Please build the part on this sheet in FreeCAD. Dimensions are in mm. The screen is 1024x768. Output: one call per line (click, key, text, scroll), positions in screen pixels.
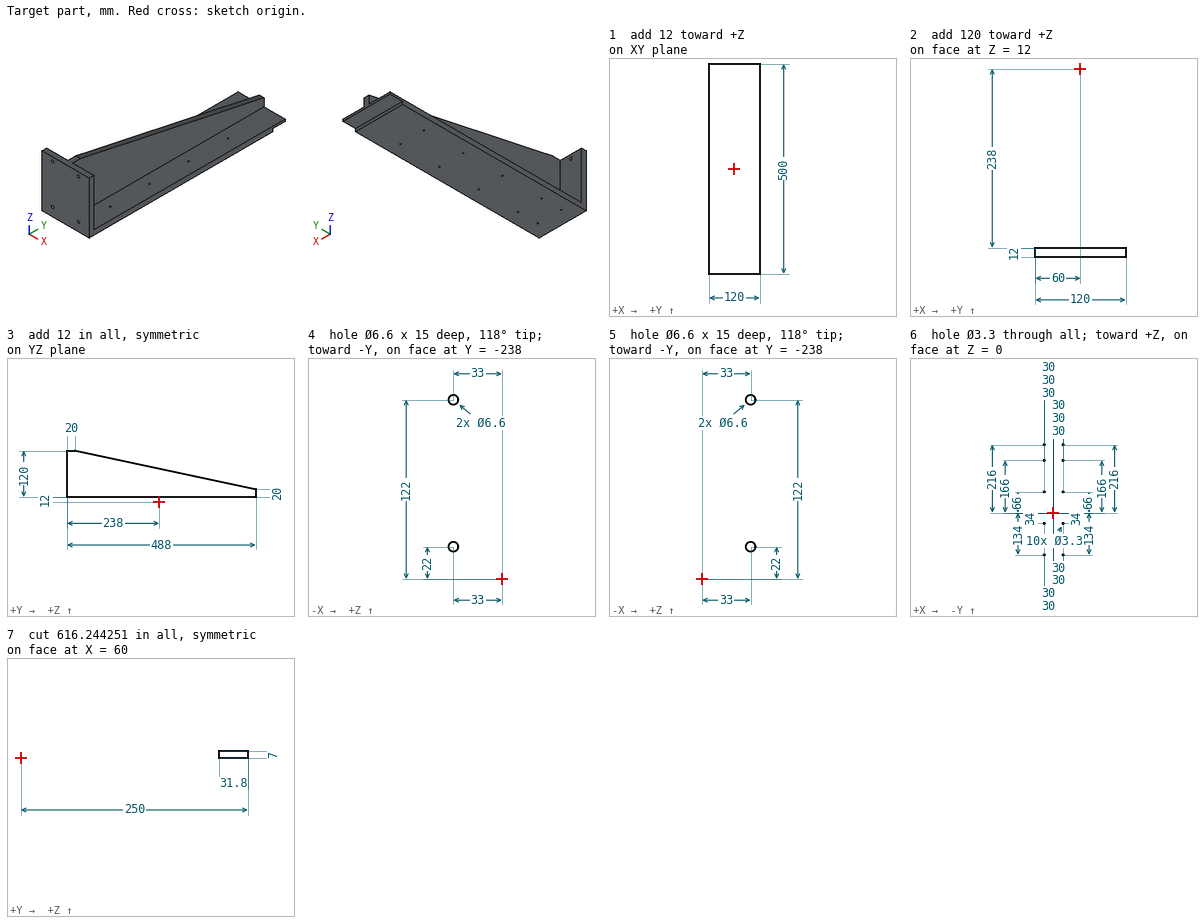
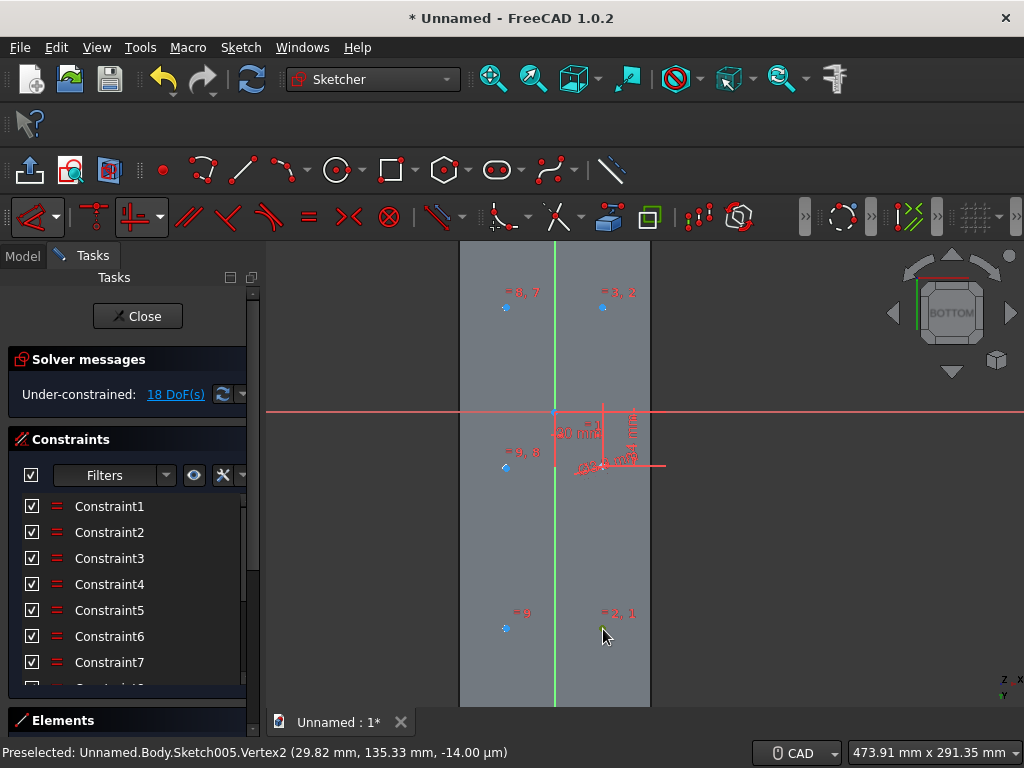
click(58, 218)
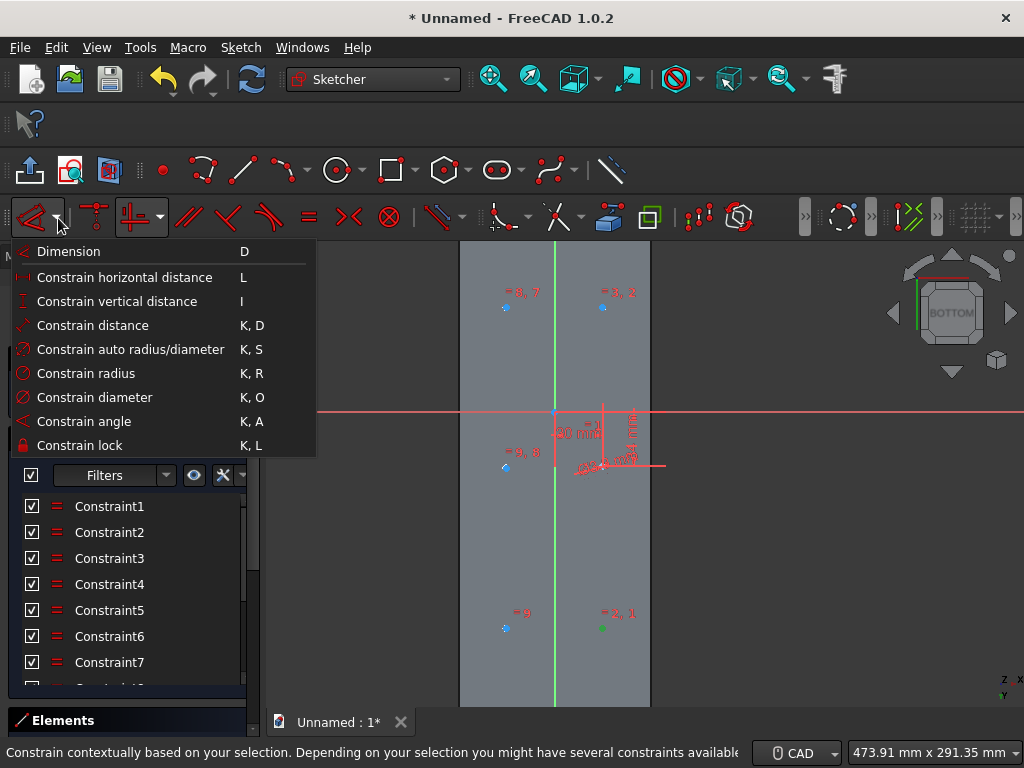
click(164, 277)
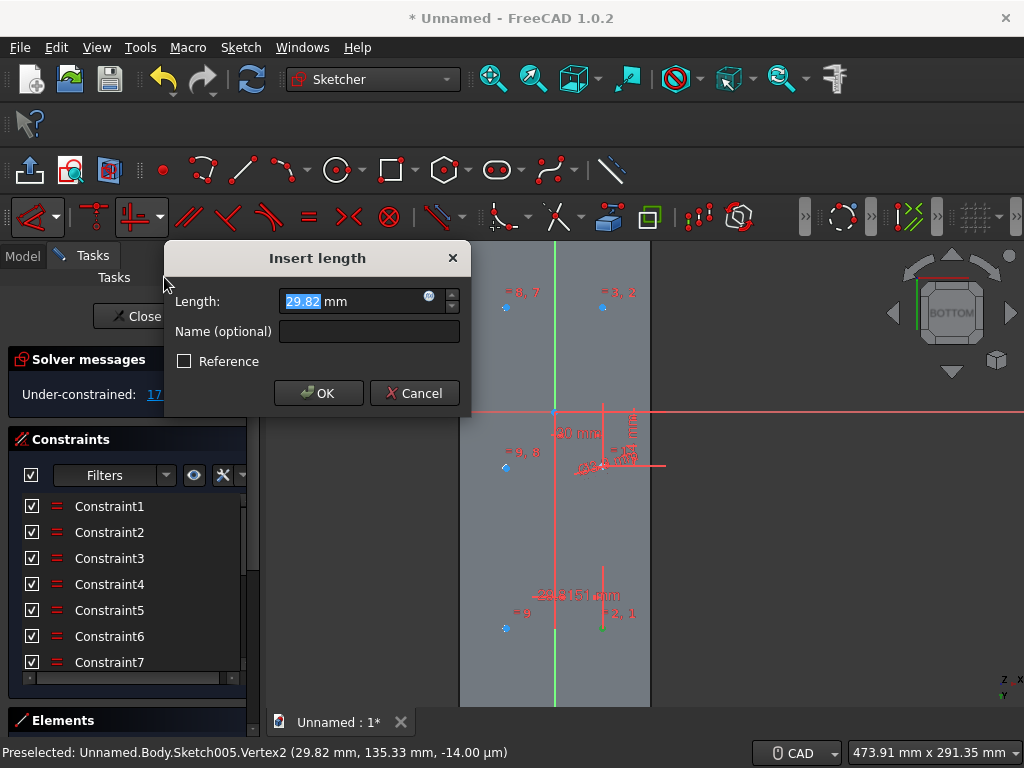
text(30)
key(Return)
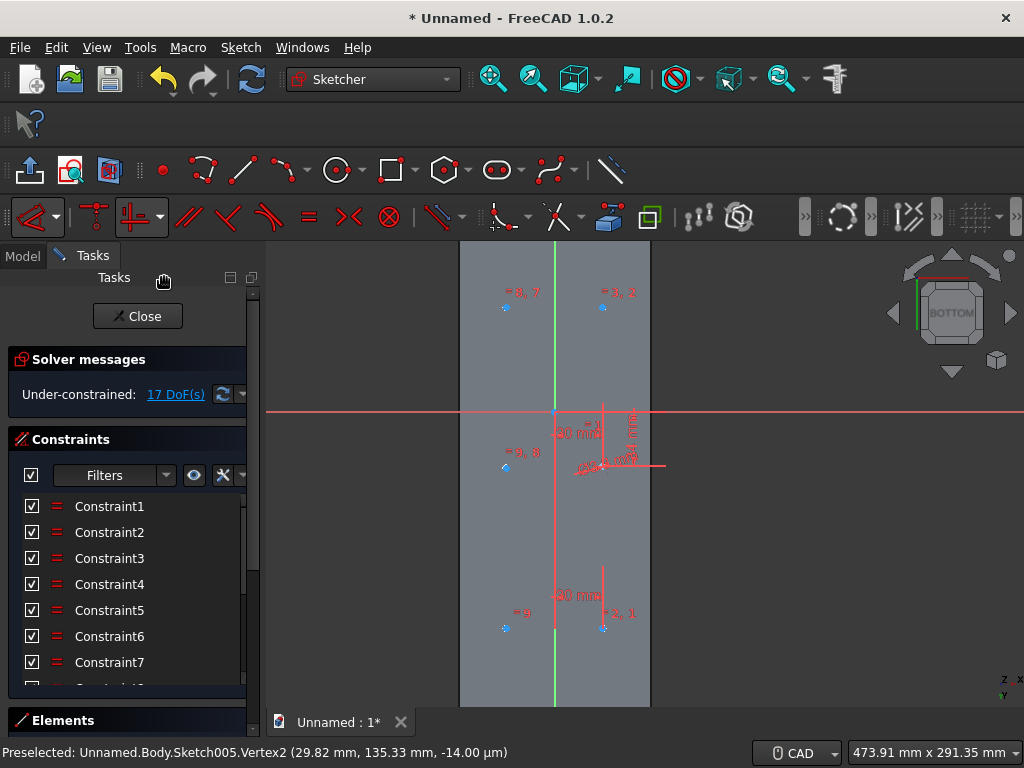
click(603, 308)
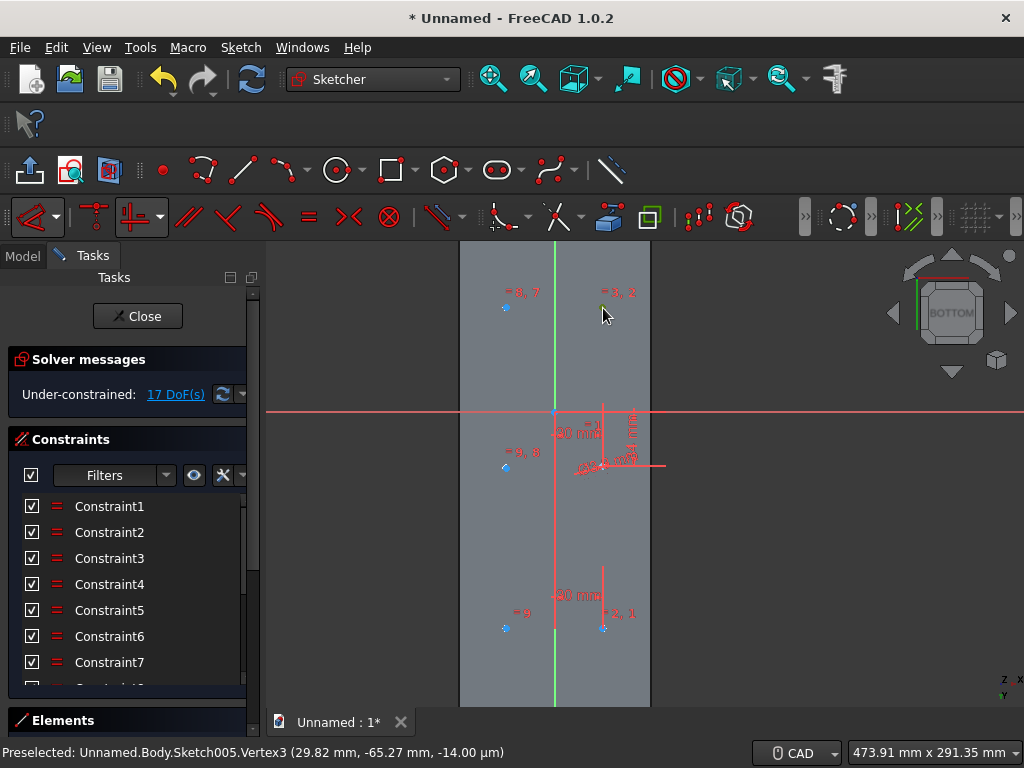
click(58, 218)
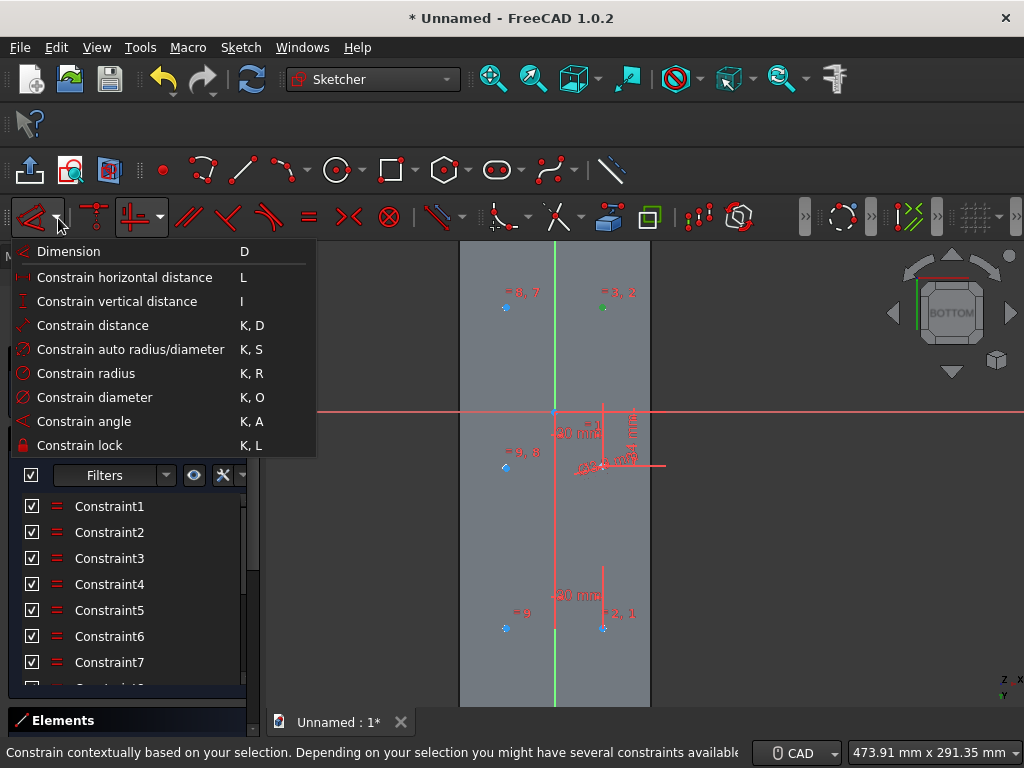
click(164, 277)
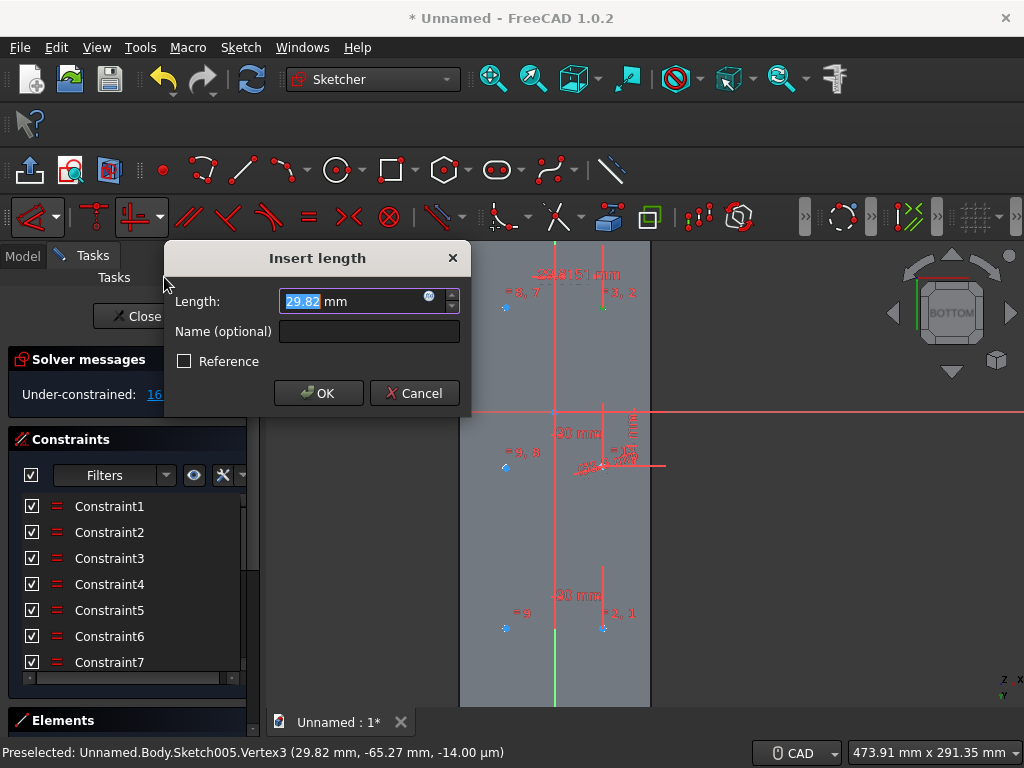
text(30)
key(Return)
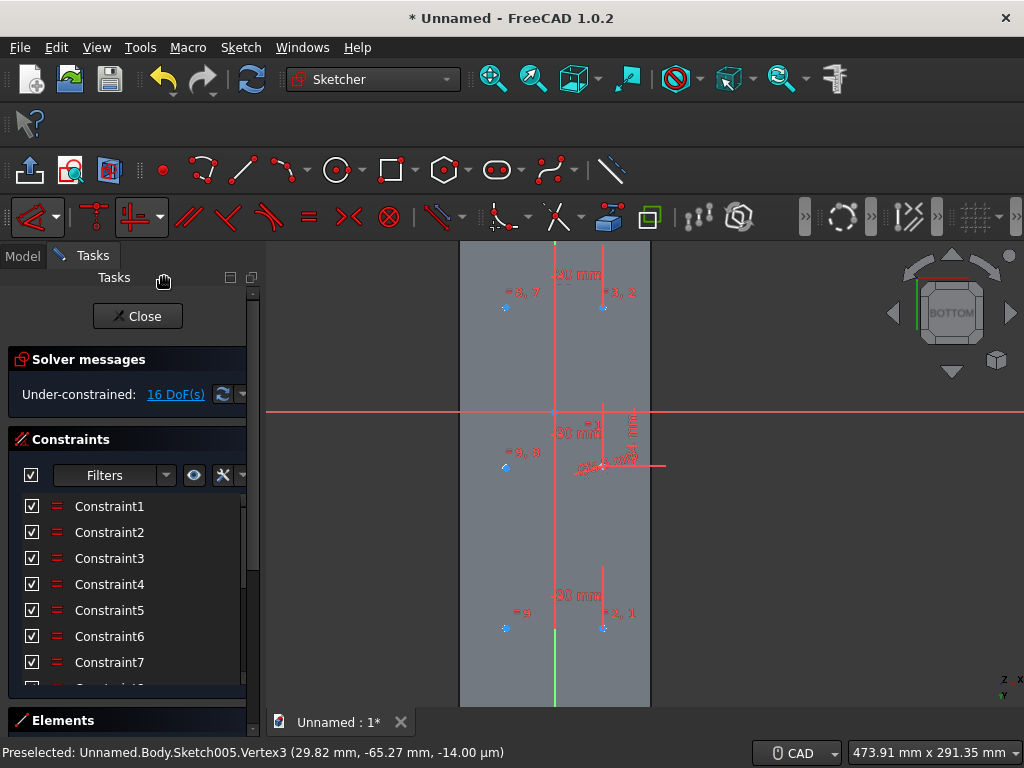
click(603, 308)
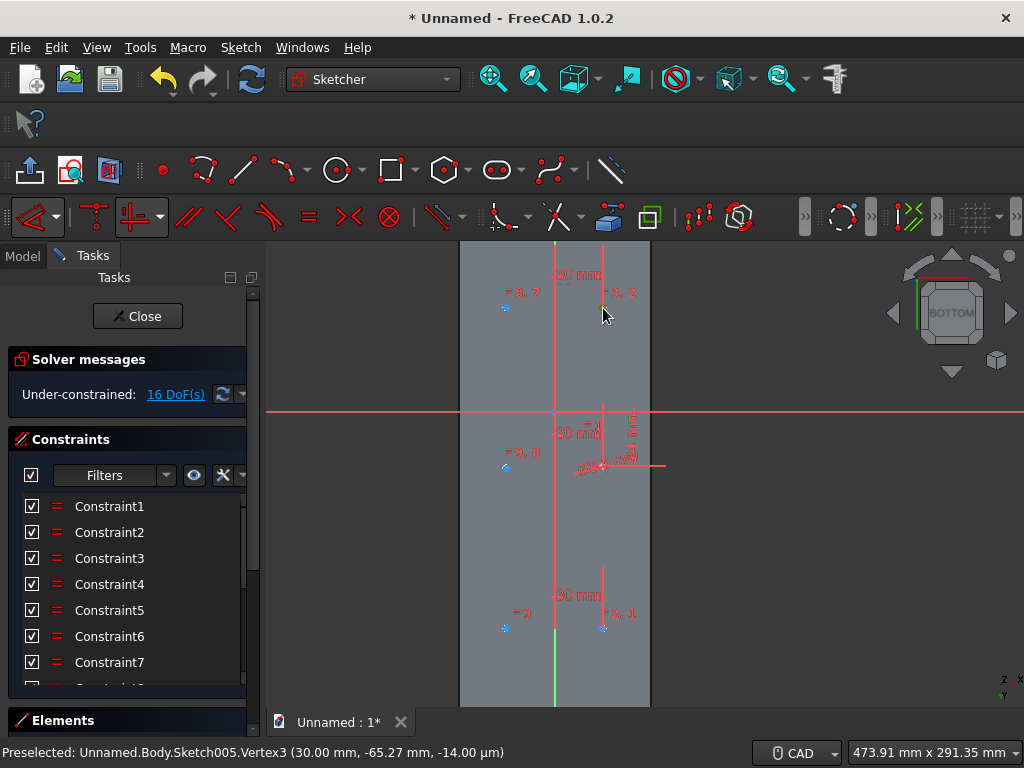
key(i)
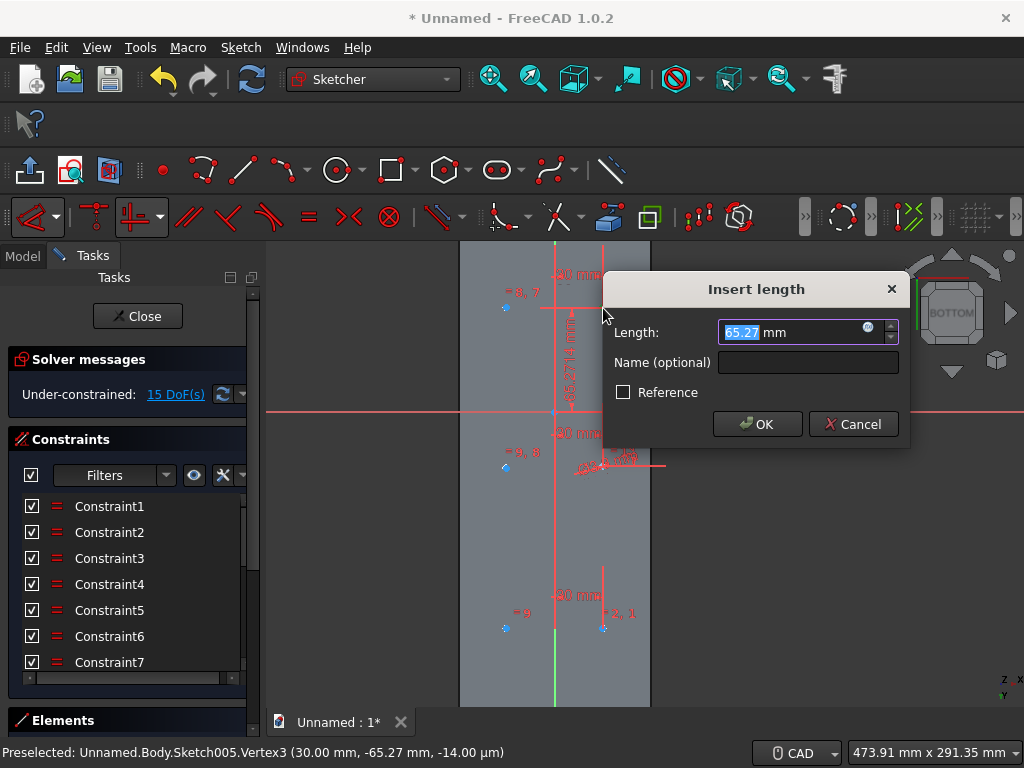
text(66)
key(Return)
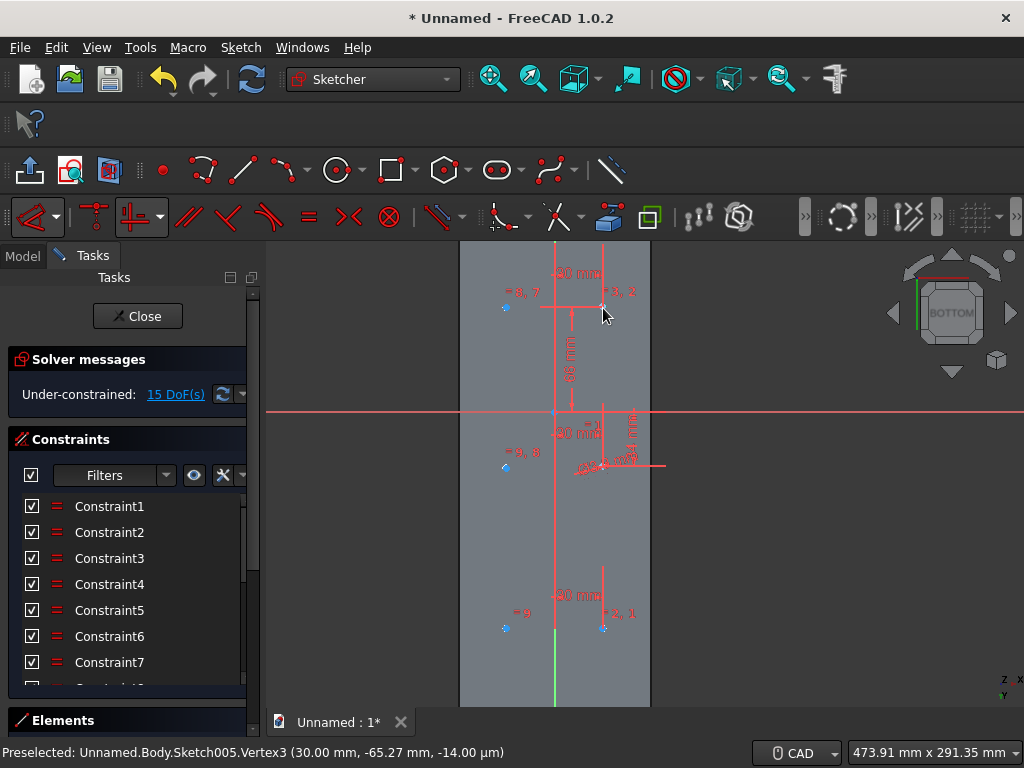
scroll(603, 629, down, 3)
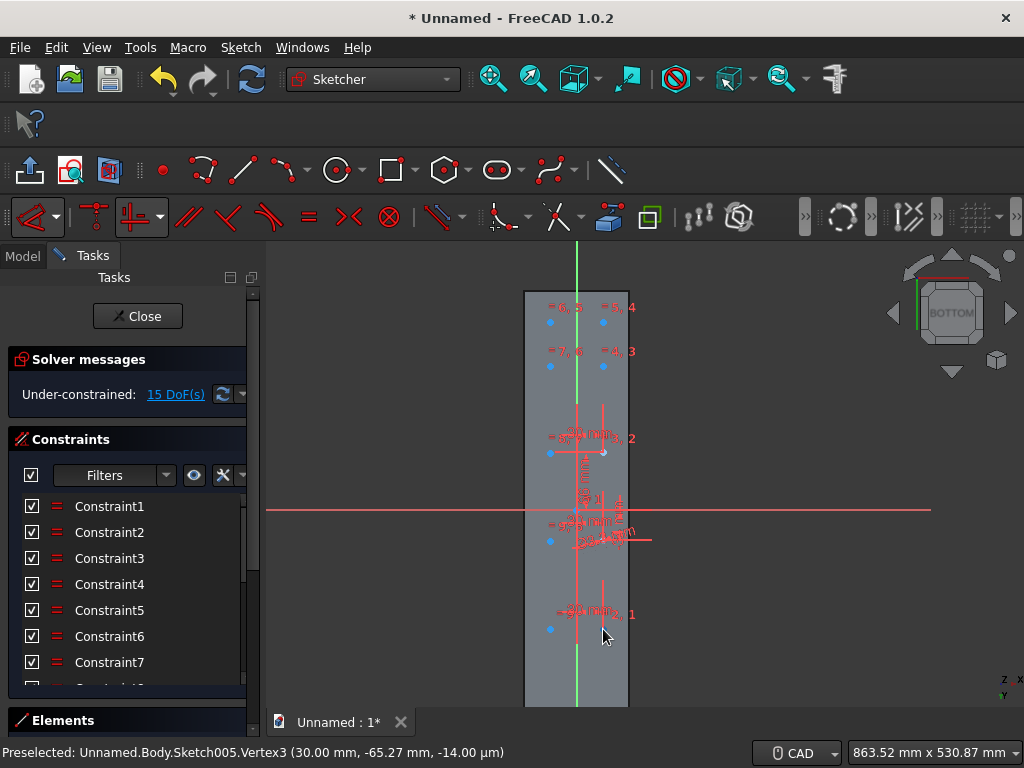
scroll(603, 366, up, 3)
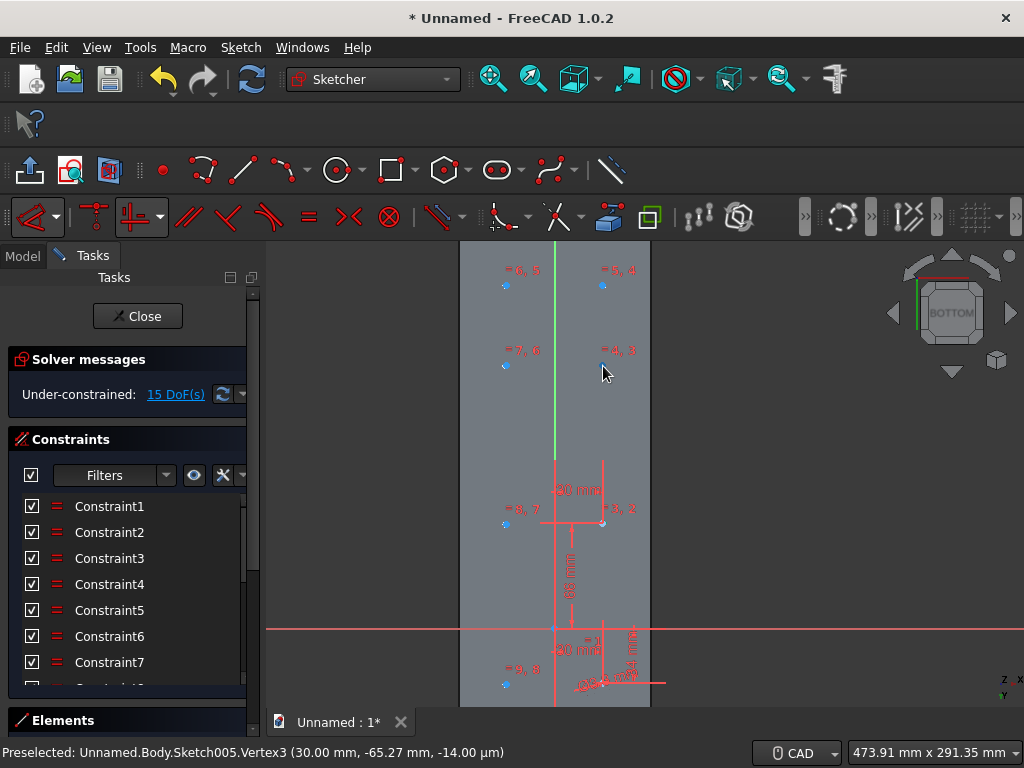
click(603, 366)